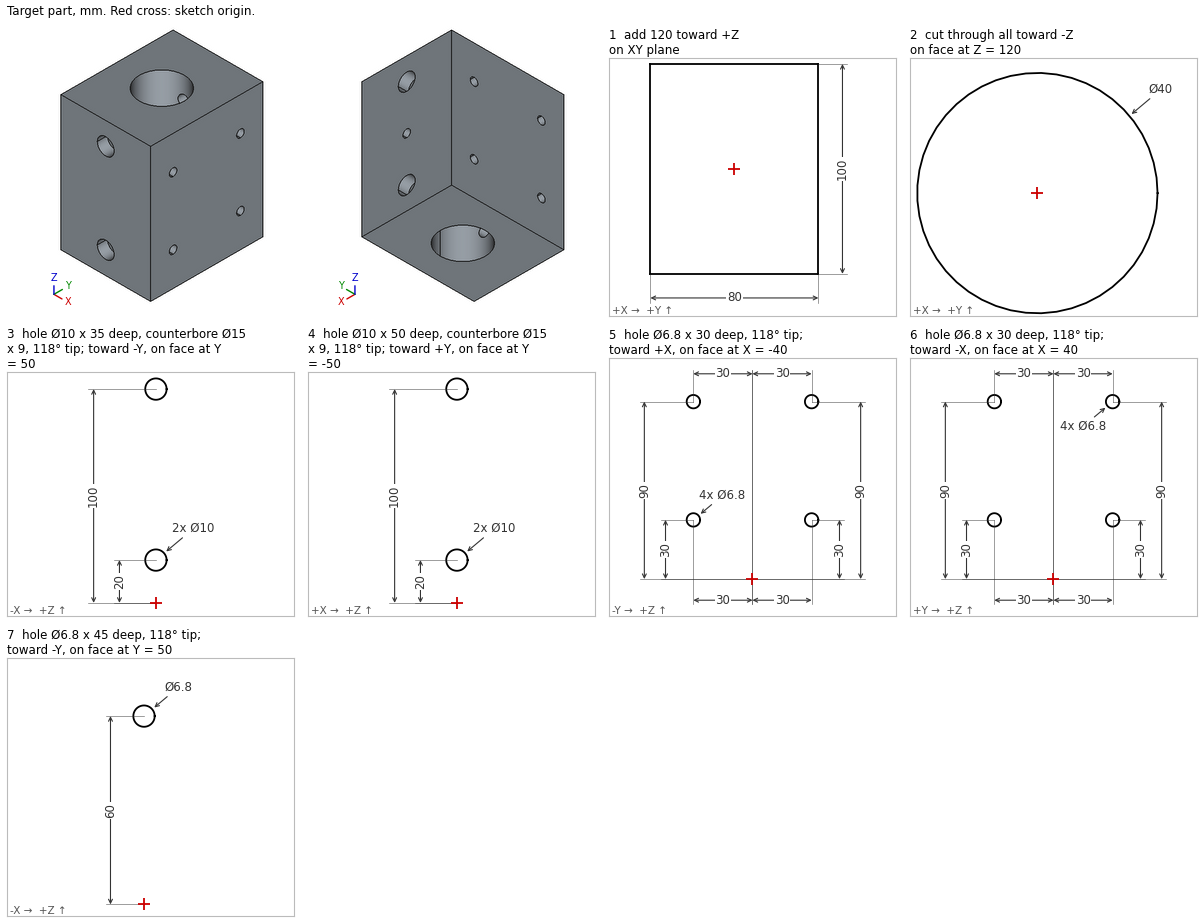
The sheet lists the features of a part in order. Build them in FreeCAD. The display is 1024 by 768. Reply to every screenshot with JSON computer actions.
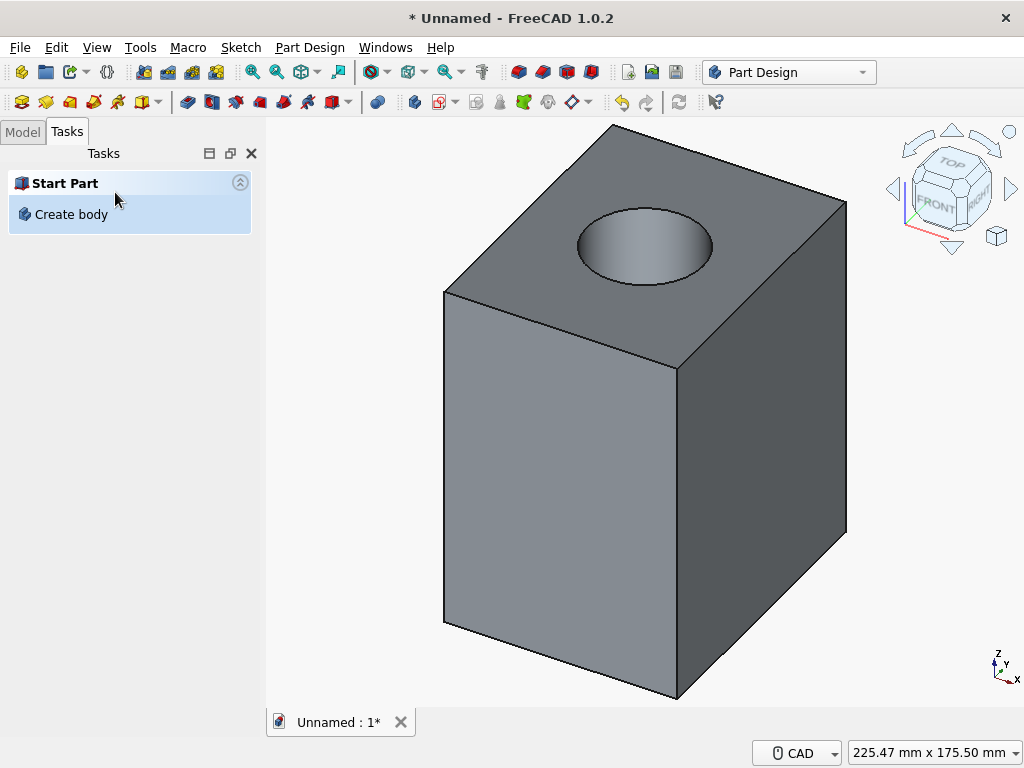
{"action": "key", "text": "4"}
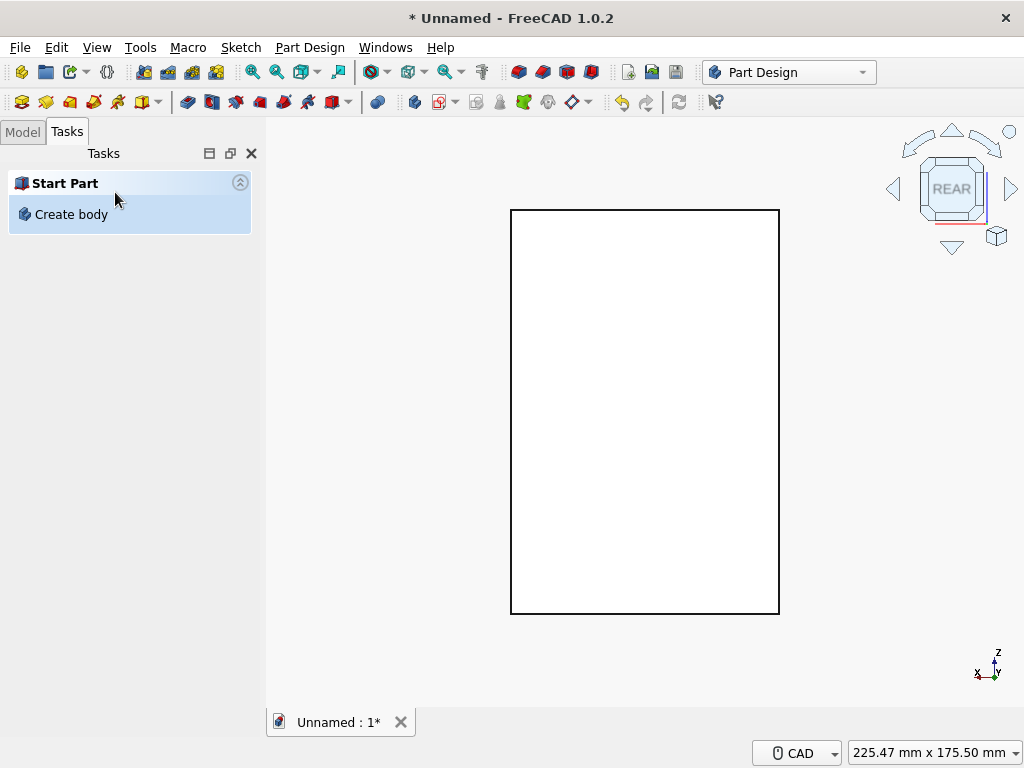
{"action": "left_click", "coordinate": [645, 353]}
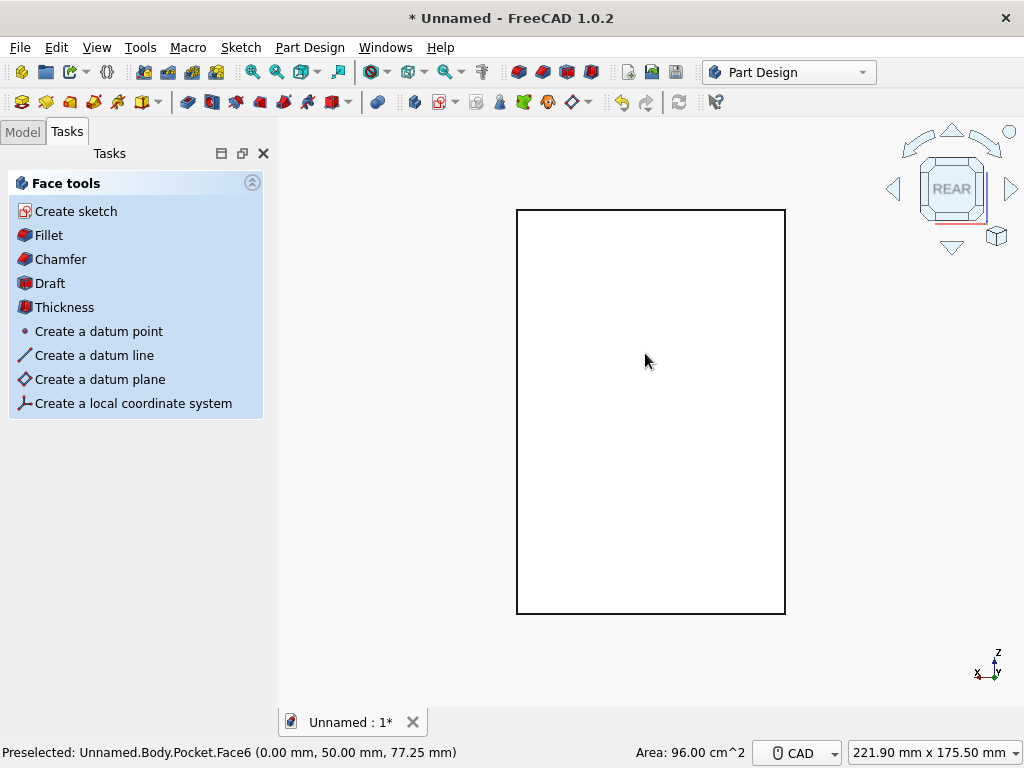
{"action": "left_click", "coordinate": [440, 102]}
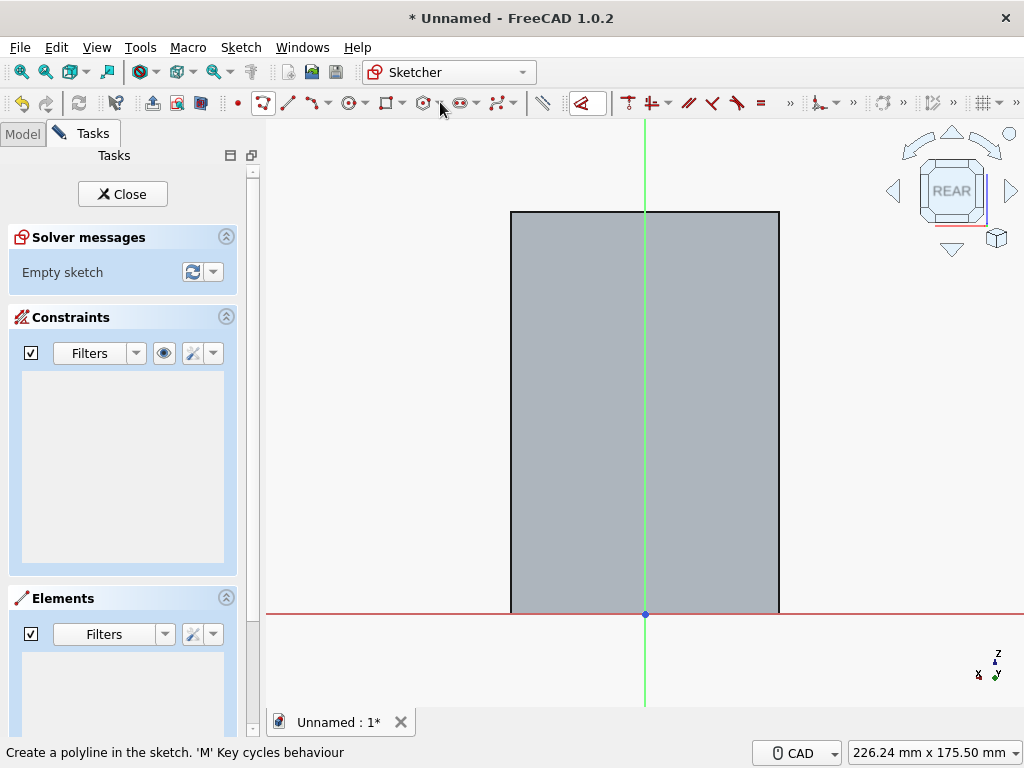
{"action": "key", "text": "g c"}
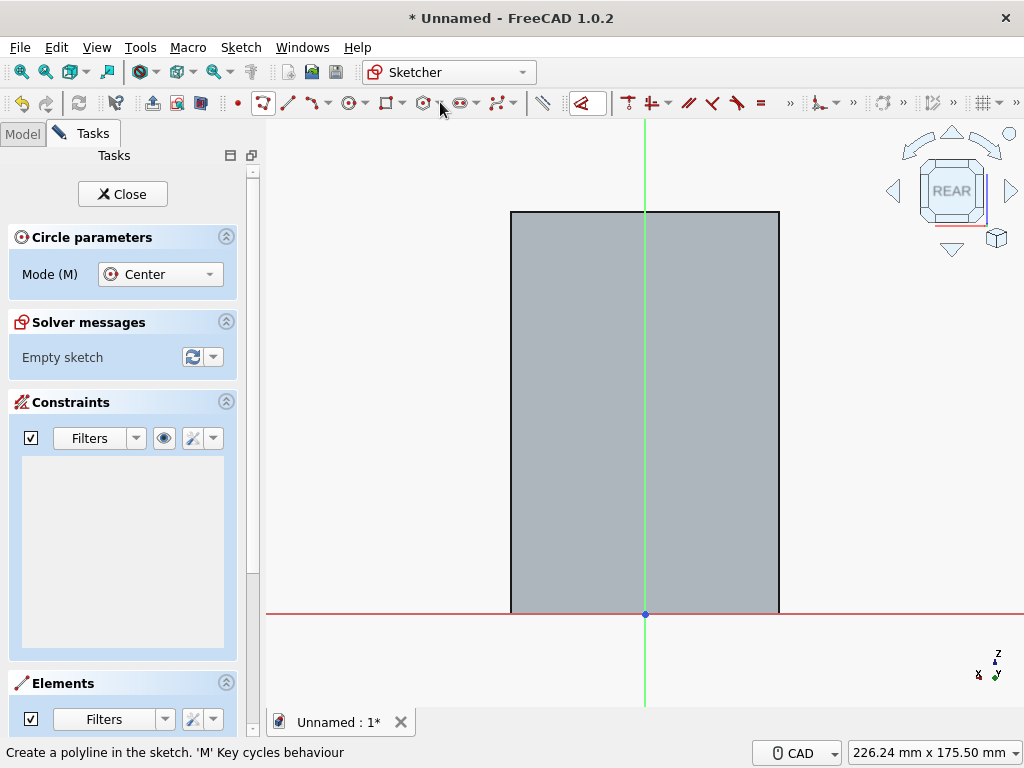
{"action": "scroll", "coordinate": [645, 547], "scroll_direction": "up", "scroll_amount": 2}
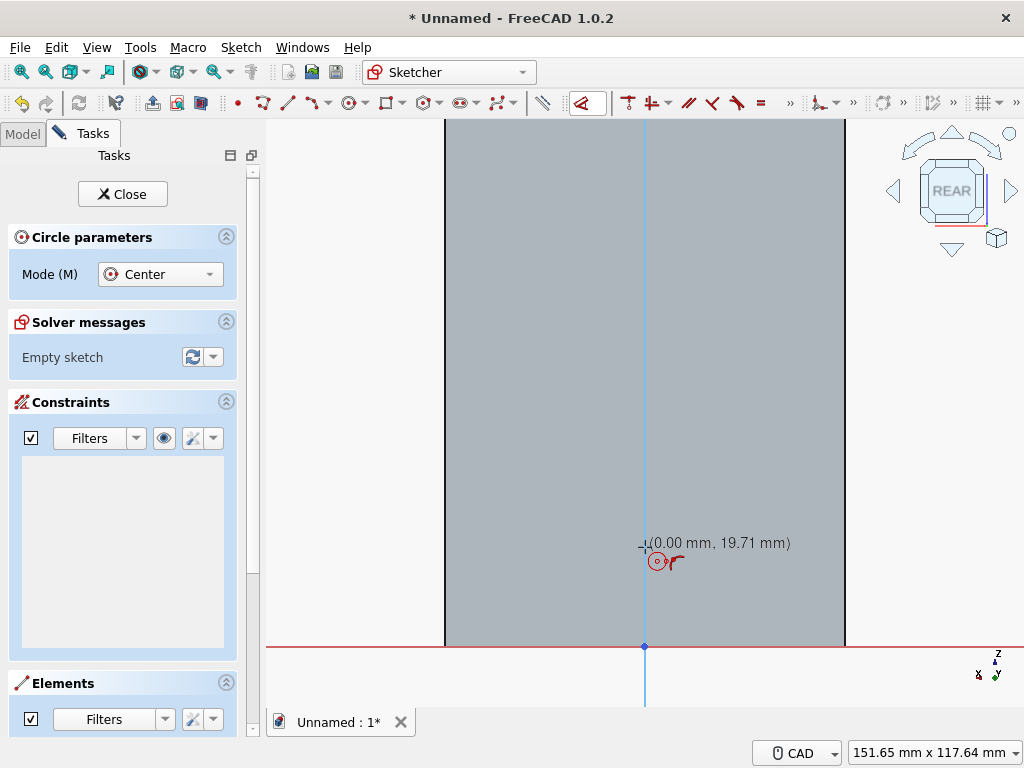
{"action": "left_click", "coordinate": [645, 547]}
{"action": "mouse_move", "coordinate": [662, 529]}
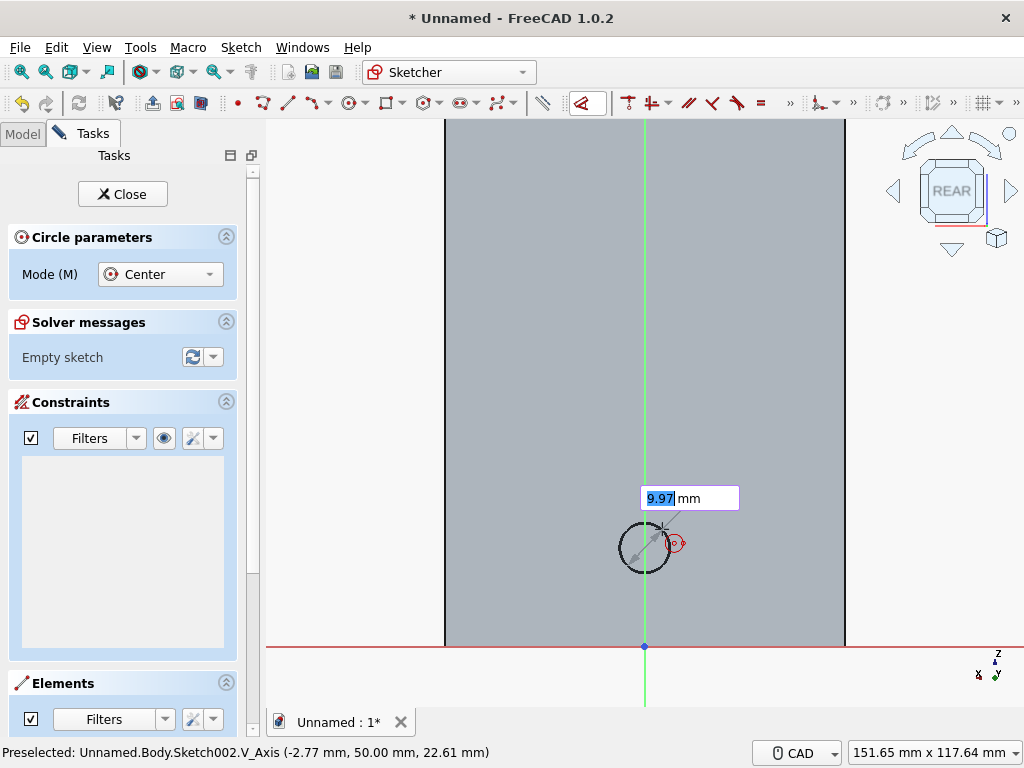
{"action": "type", "text": "10"}
{"action": "key", "text": "Return"}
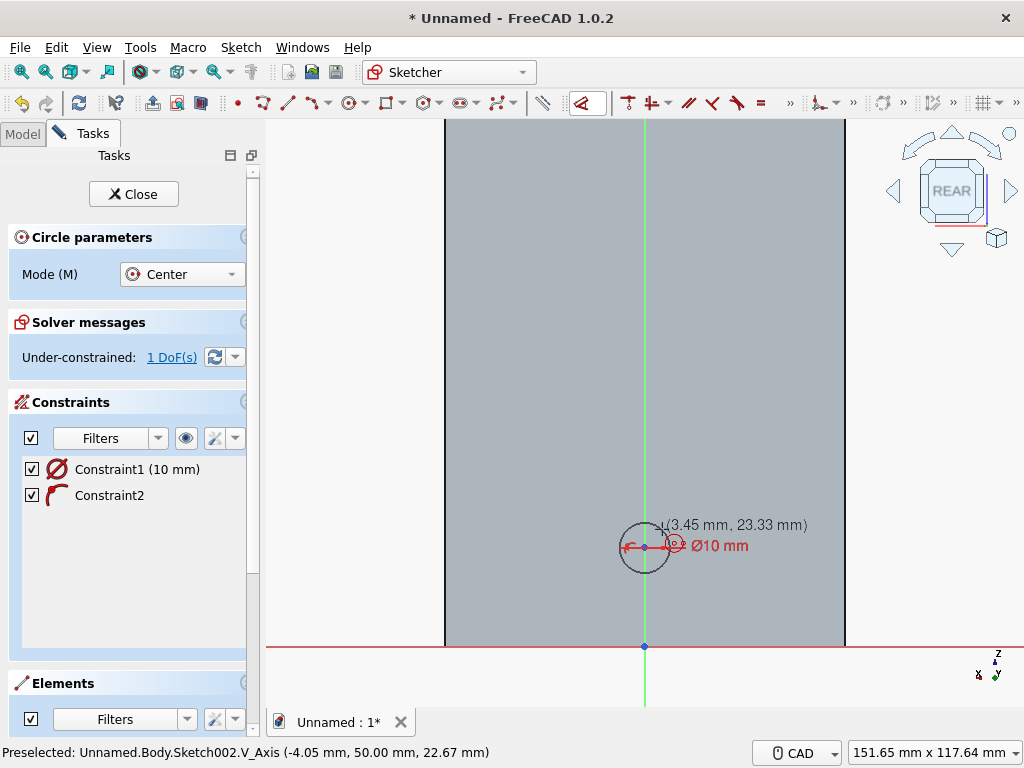
{"action": "scroll", "coordinate": [438, 472], "scroll_direction": "down", "scroll_amount": 2}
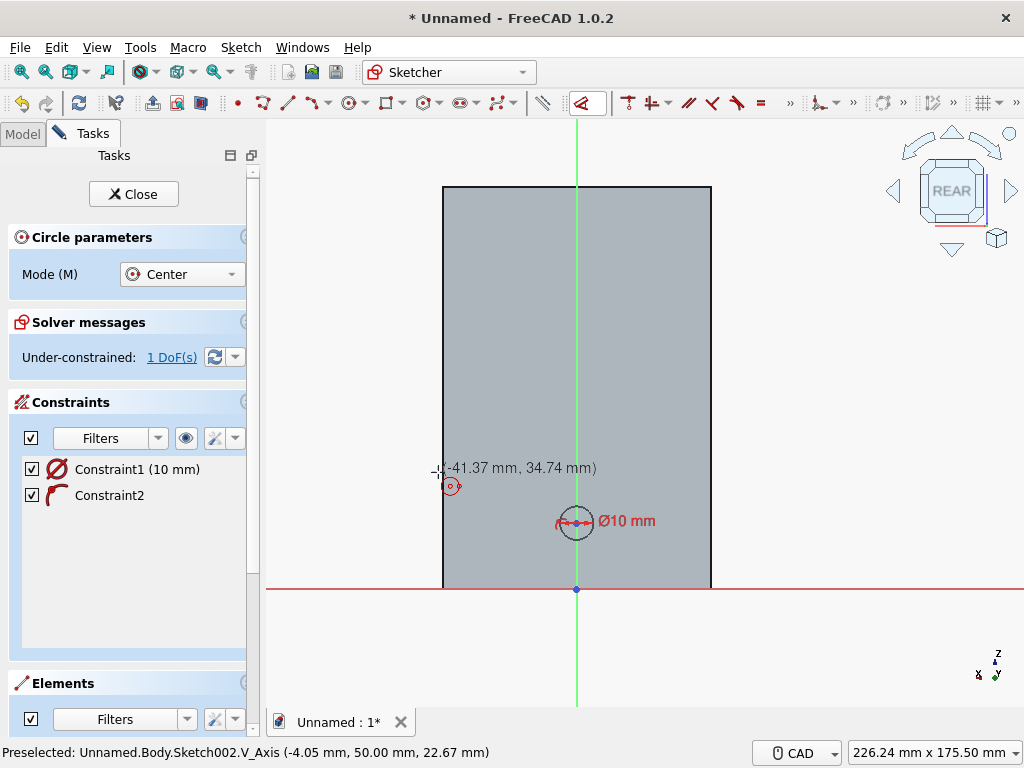
{"action": "scroll", "coordinate": [577, 254], "scroll_direction": "up", "scroll_amount": 2}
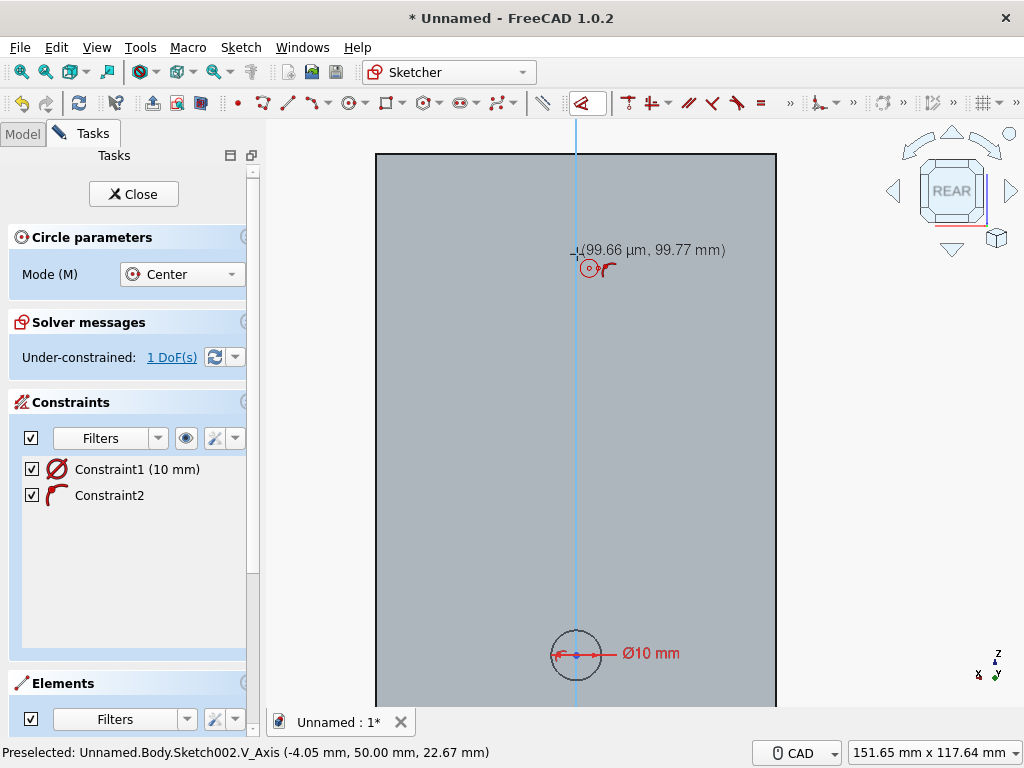
{"action": "left_click", "coordinate": [576, 254]}
{"action": "mouse_move", "coordinate": [594, 237]}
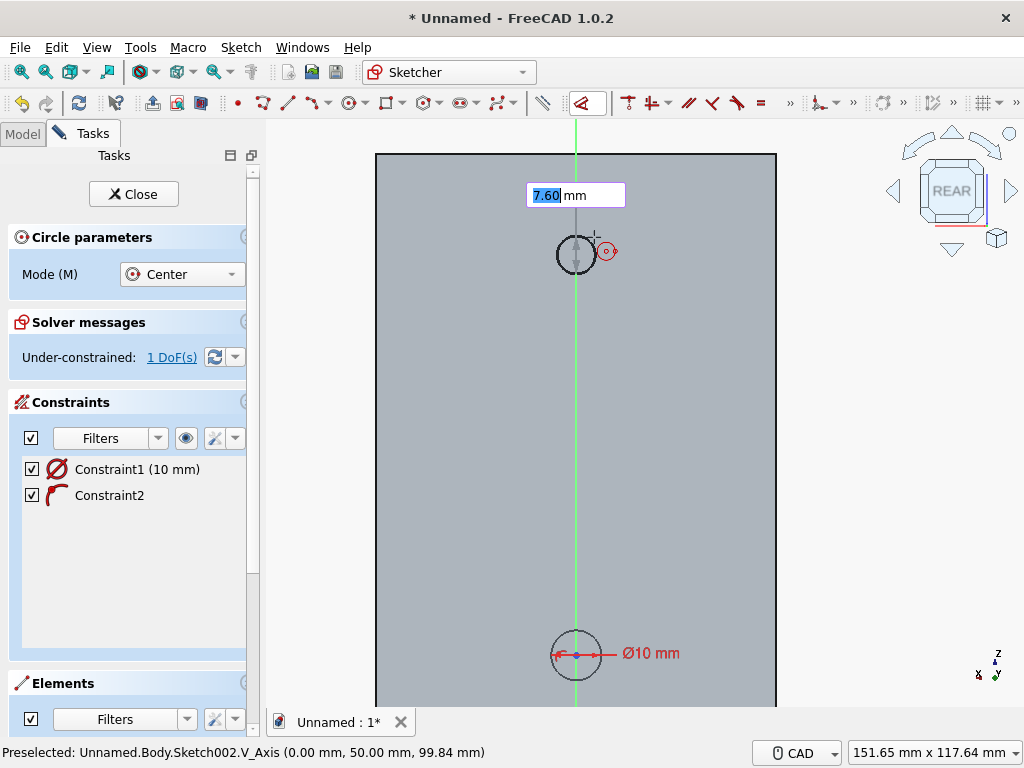
{"action": "type", "text": "10"}
{"action": "key", "text": "Return"}
{"action": "key", "text": "Escape"}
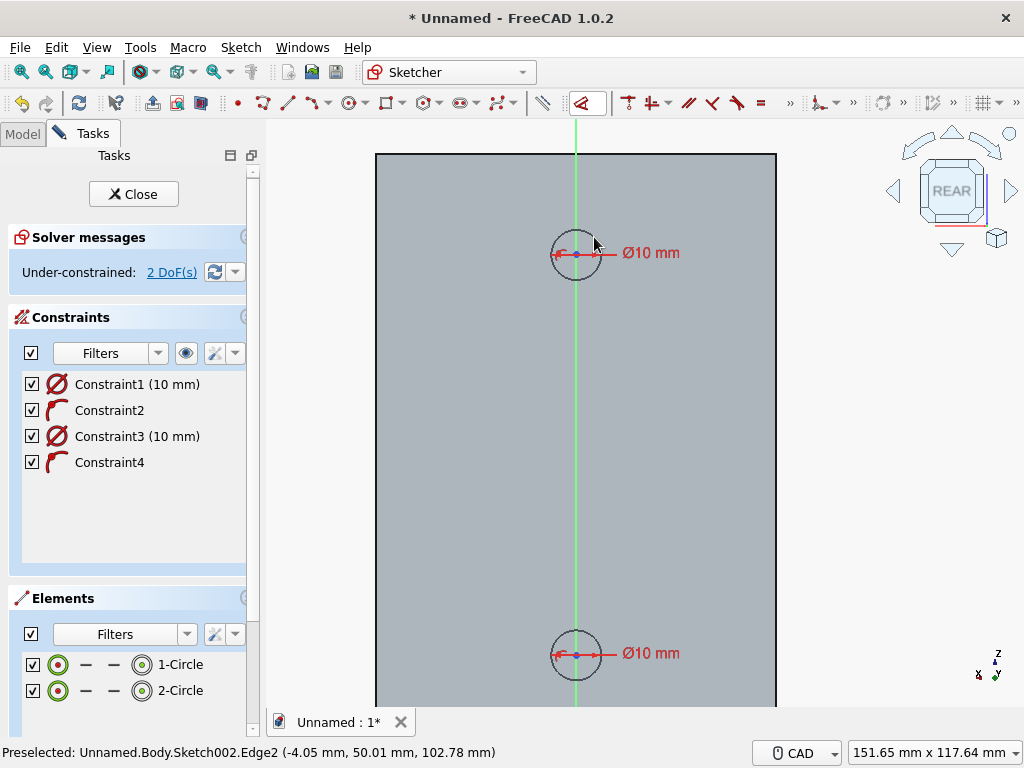
{"action": "left_click", "coordinate": [582, 104]}